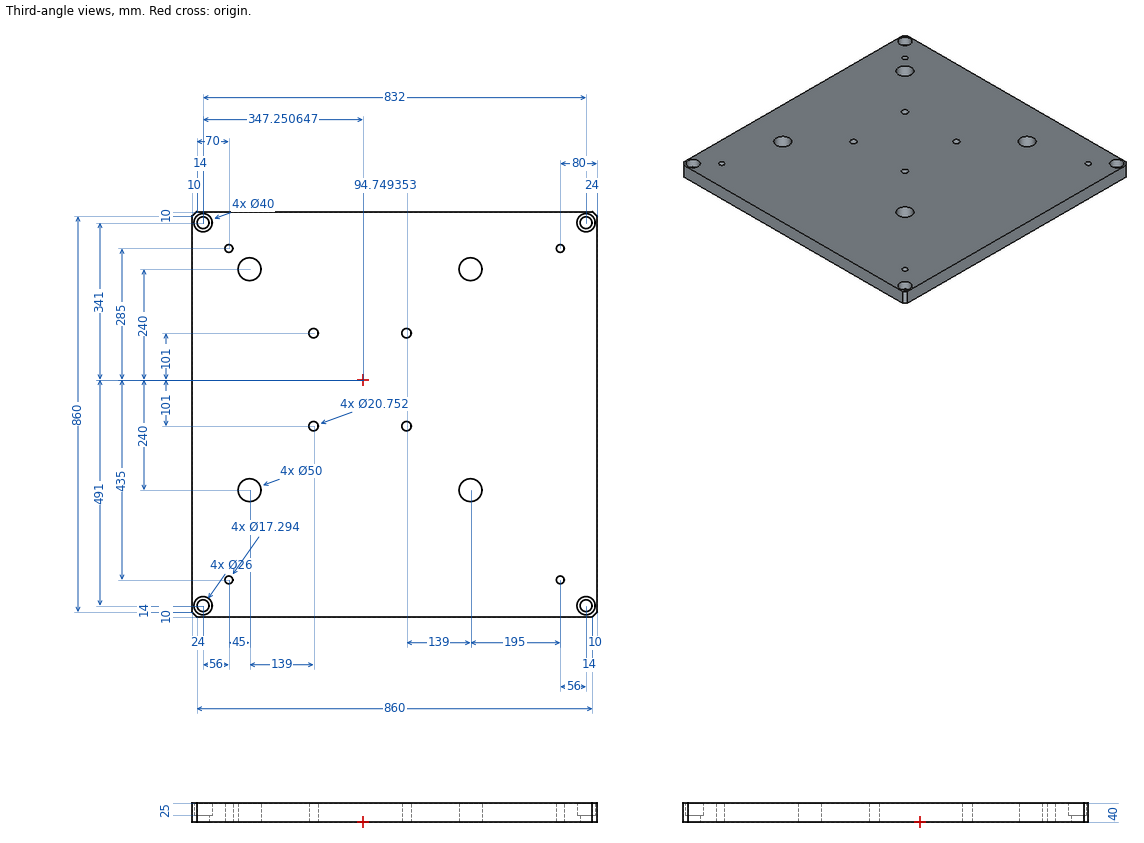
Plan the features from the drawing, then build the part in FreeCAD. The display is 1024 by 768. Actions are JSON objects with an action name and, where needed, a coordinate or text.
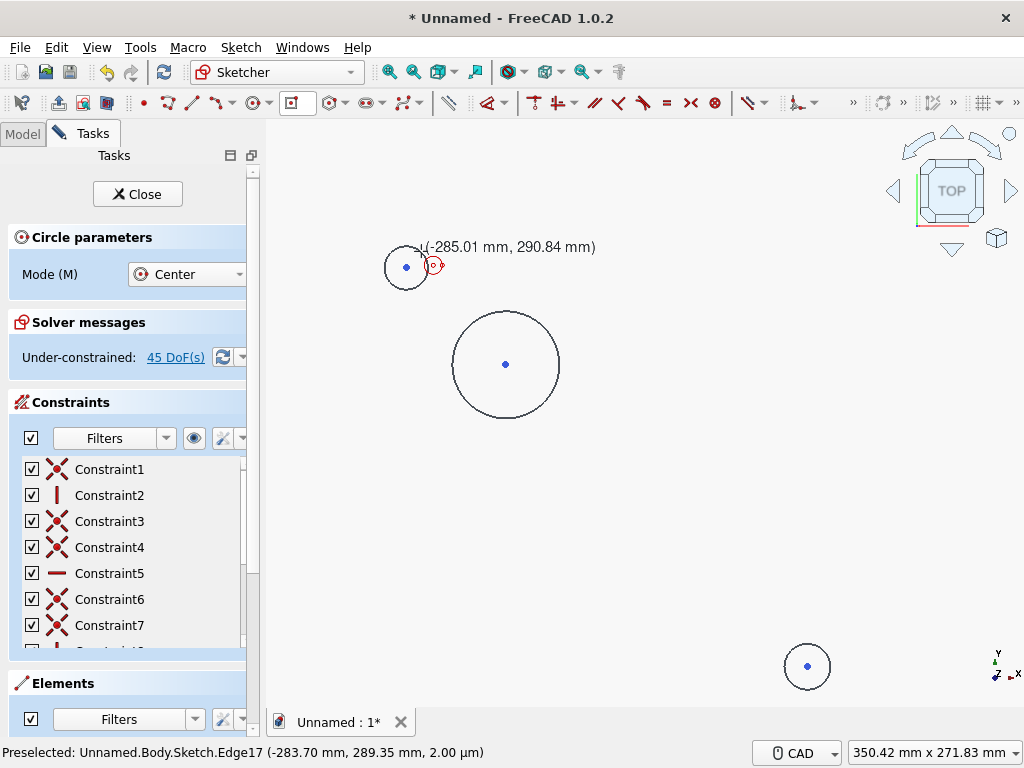
{"action": "scroll", "coordinate": [422, 254], "scroll_direction": "down", "scroll_amount": 8}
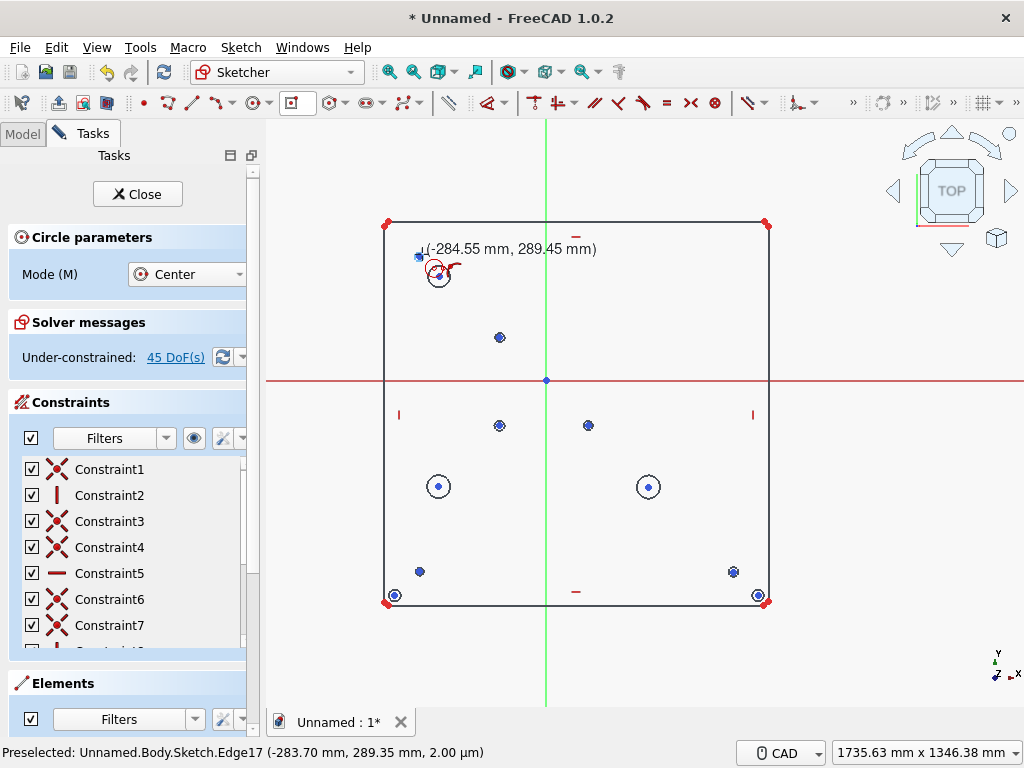
{"action": "scroll", "coordinate": [395, 232], "scroll_direction": "up", "scroll_amount": 7}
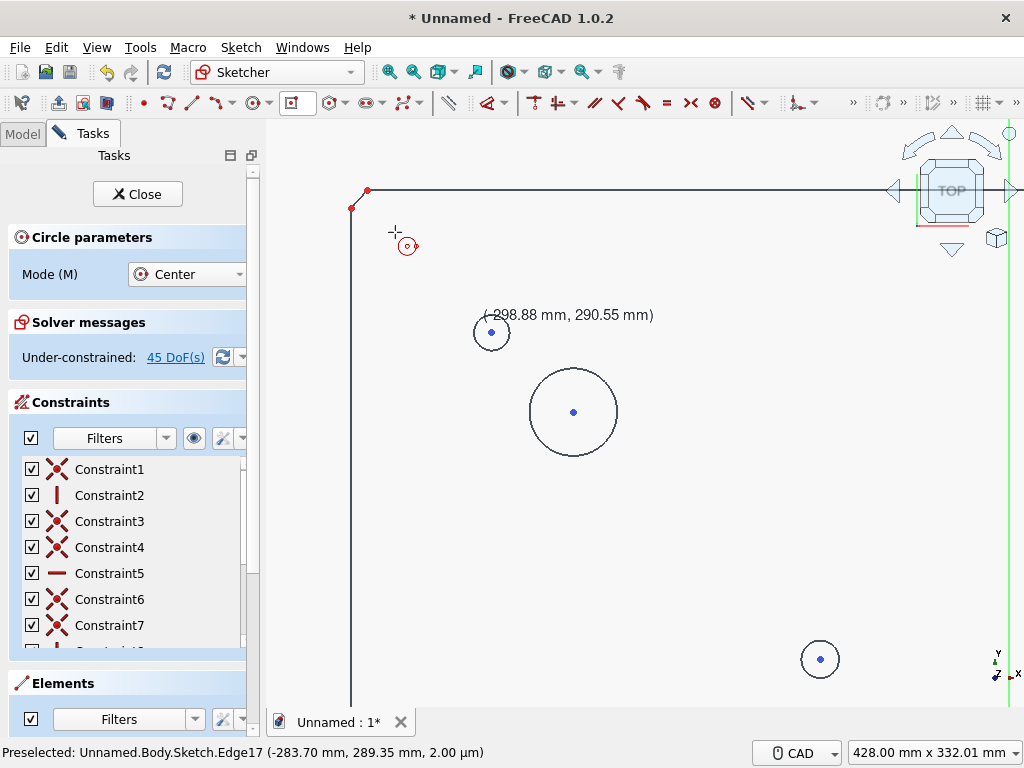
{"action": "left_click", "coordinate": [394, 231]}
{"action": "left_click", "coordinate": [410, 215]}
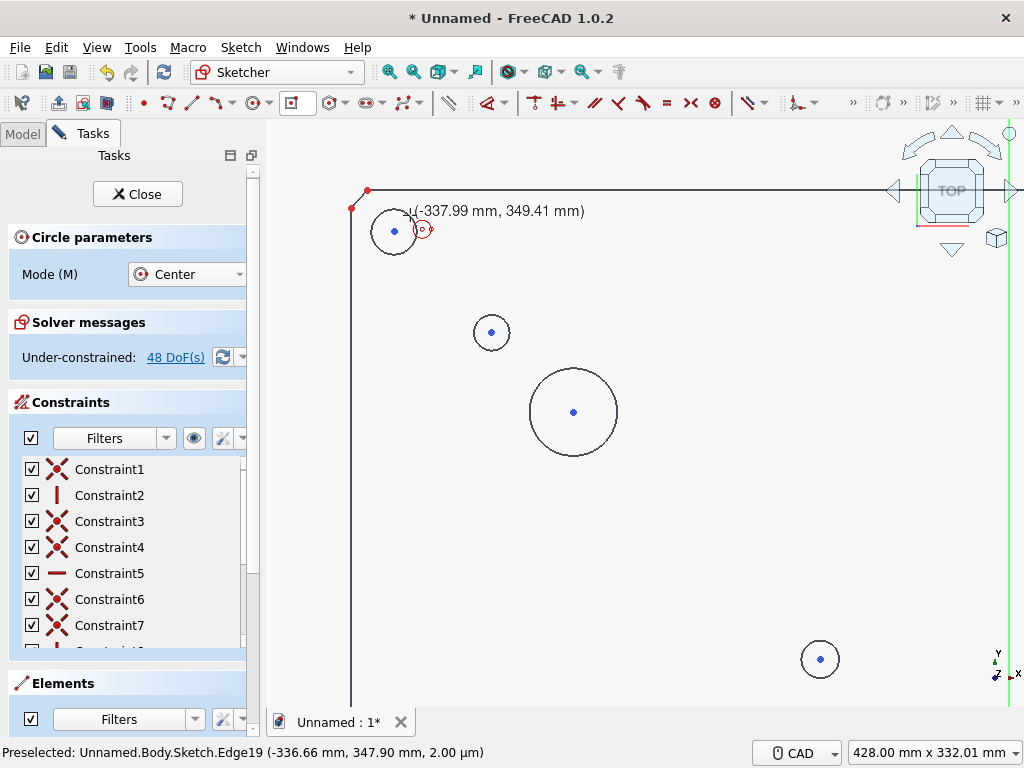
{"action": "scroll", "coordinate": [395, 231], "scroll_direction": "down", "scroll_amount": 7}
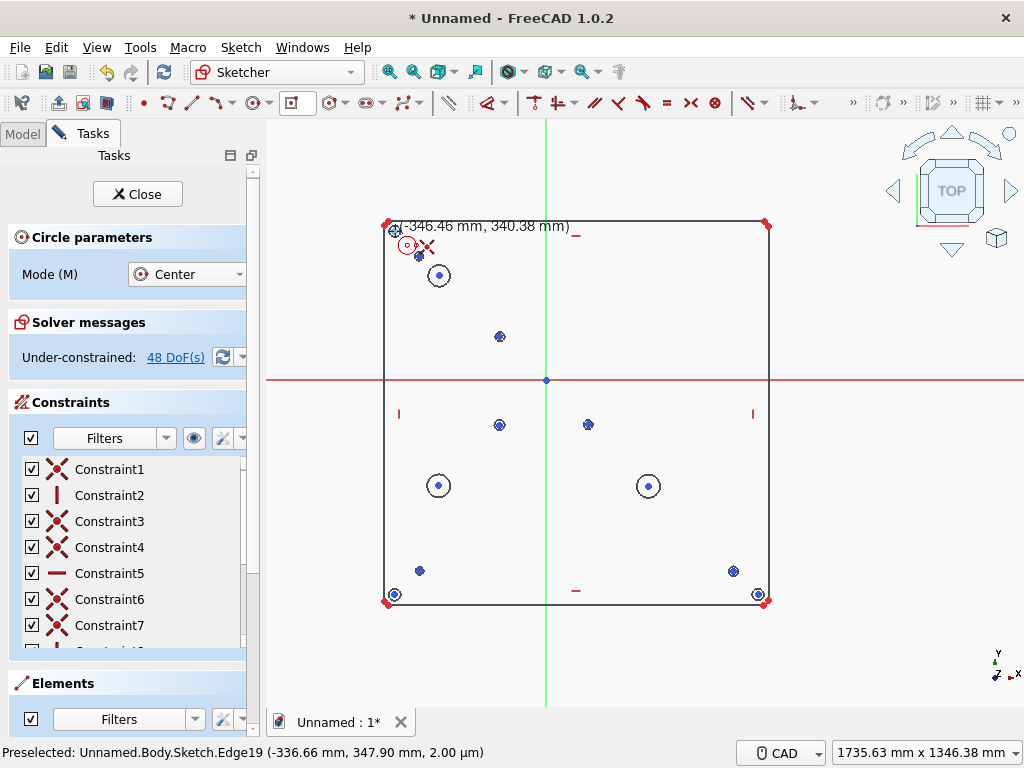
{"action": "scroll", "coordinate": [588, 336], "scroll_direction": "up", "scroll_amount": 9}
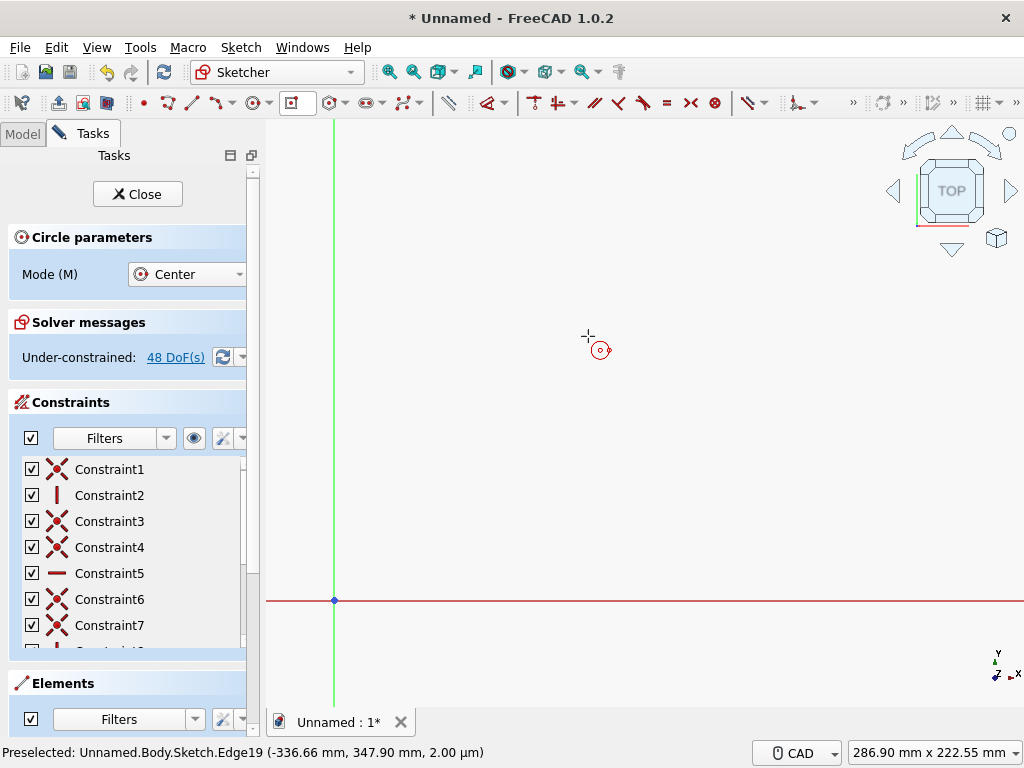
{"action": "scroll", "coordinate": [588, 337], "scroll_direction": "down", "scroll_amount": 9}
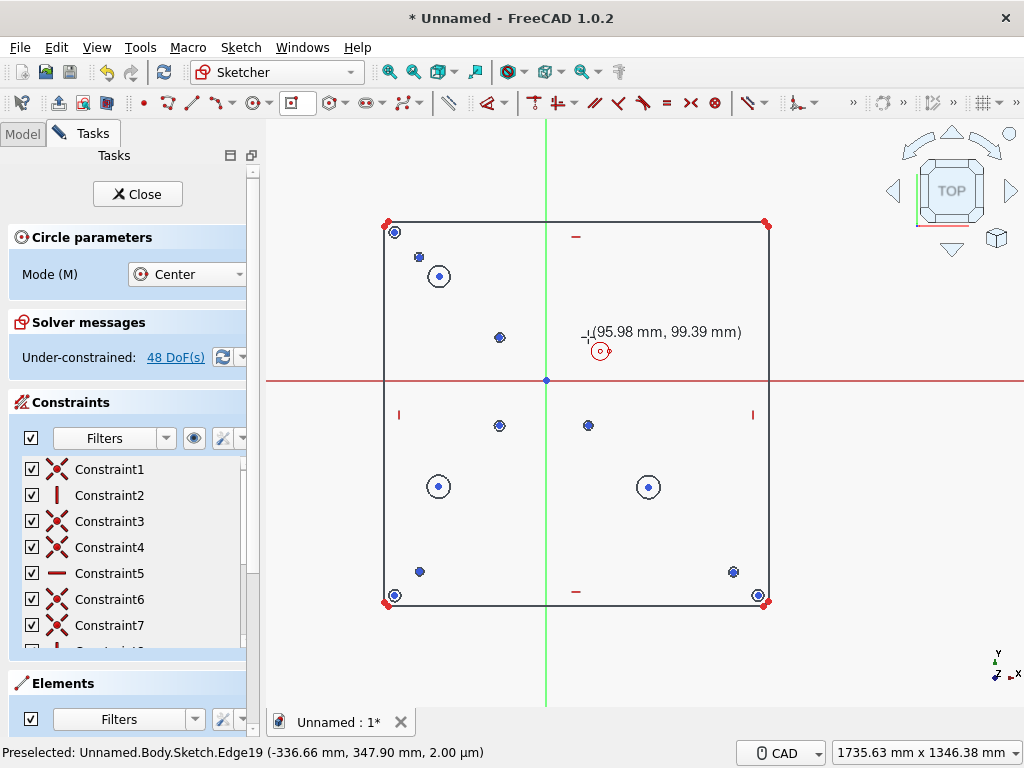
{"action": "left_click", "coordinate": [588, 337]}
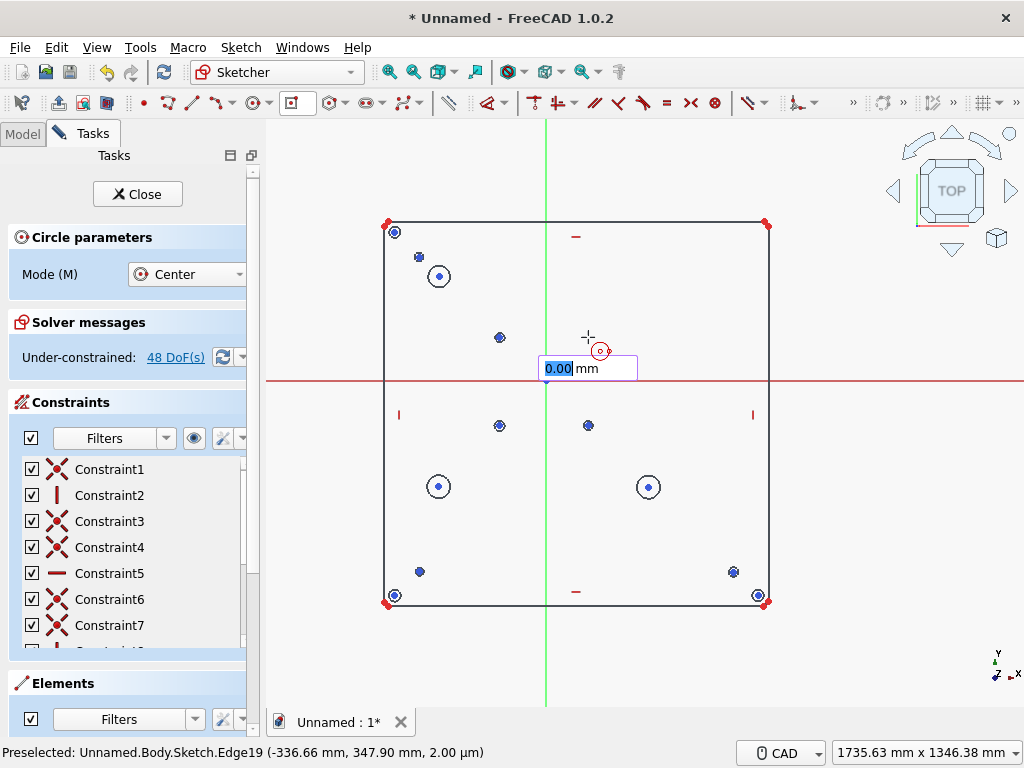
{"action": "scroll", "coordinate": [591, 334], "scroll_direction": "up", "scroll_amount": 7}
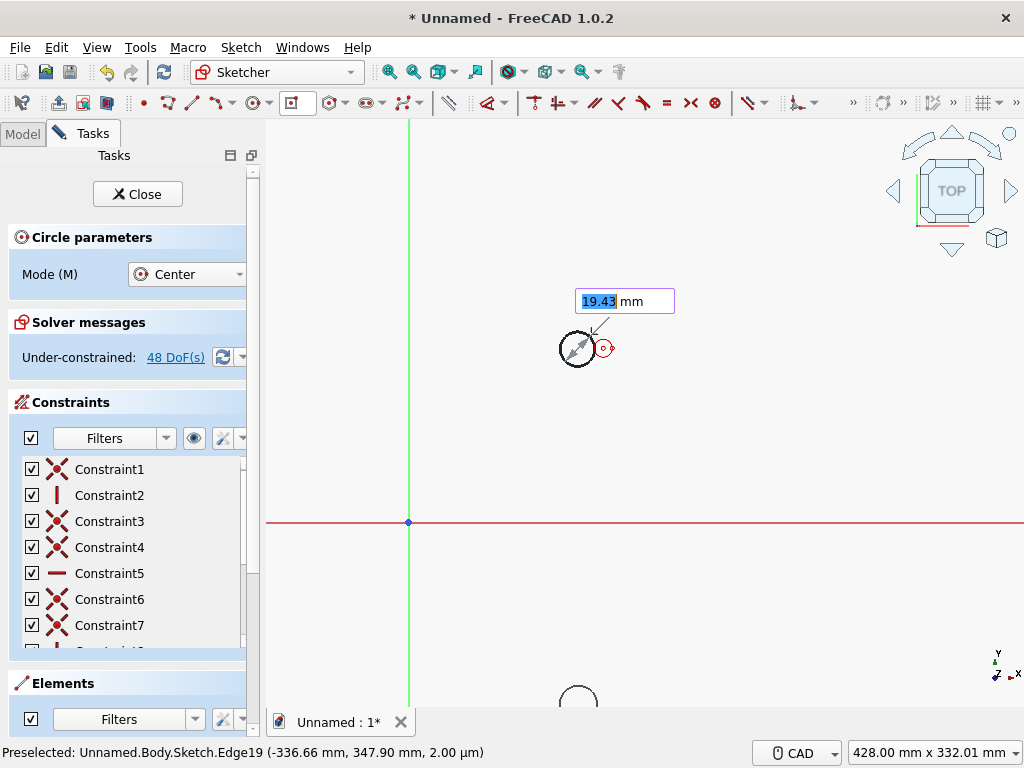
{"action": "left_click", "coordinate": [590, 331]}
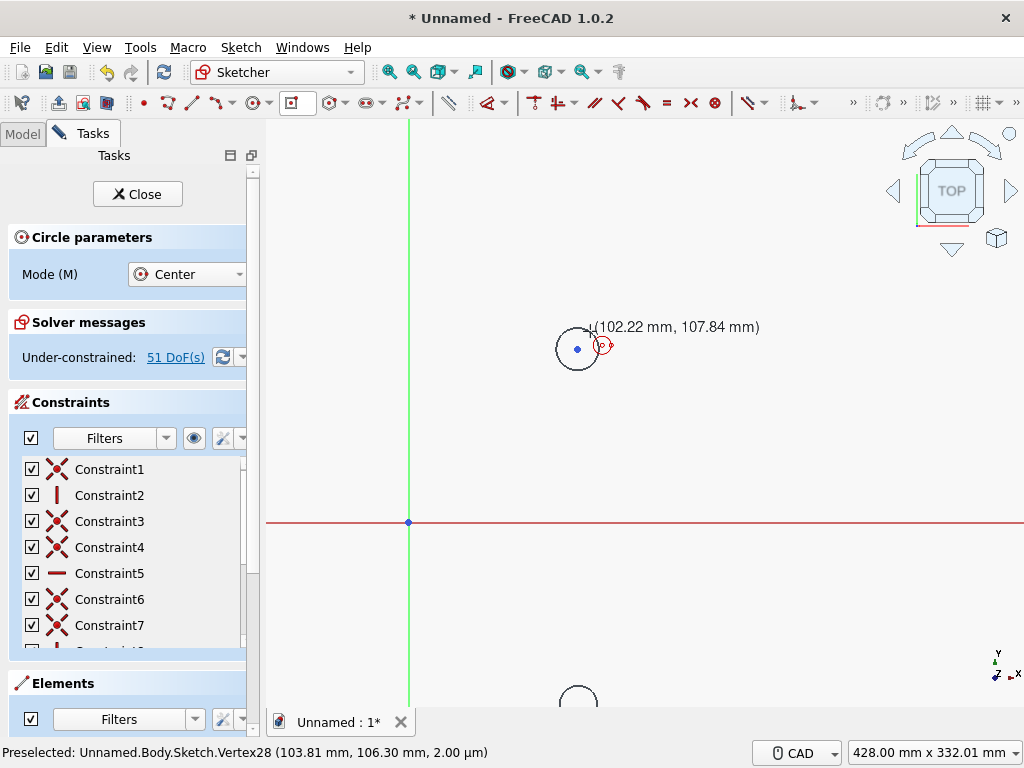
{"action": "scroll", "coordinate": [591, 334], "scroll_direction": "down", "scroll_amount": 7}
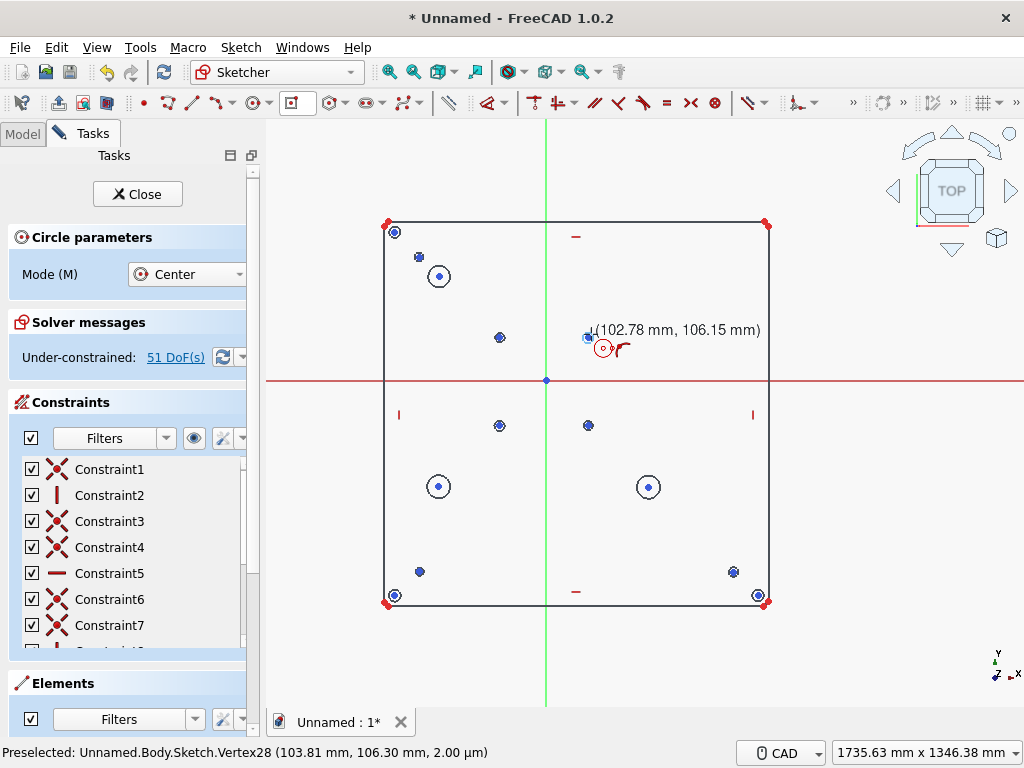
{"action": "scroll", "coordinate": [649, 276], "scroll_direction": "up", "scroll_amount": 4}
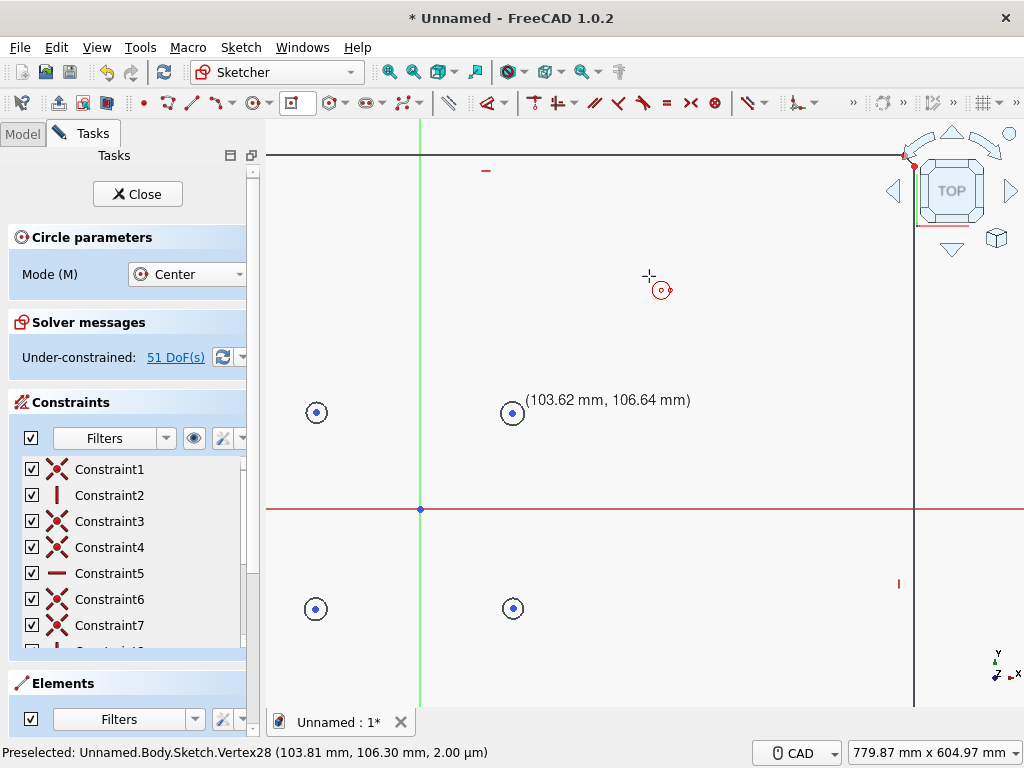
{"action": "left_click", "coordinate": [647, 276]}
{"action": "left_click", "coordinate": [664, 259]}